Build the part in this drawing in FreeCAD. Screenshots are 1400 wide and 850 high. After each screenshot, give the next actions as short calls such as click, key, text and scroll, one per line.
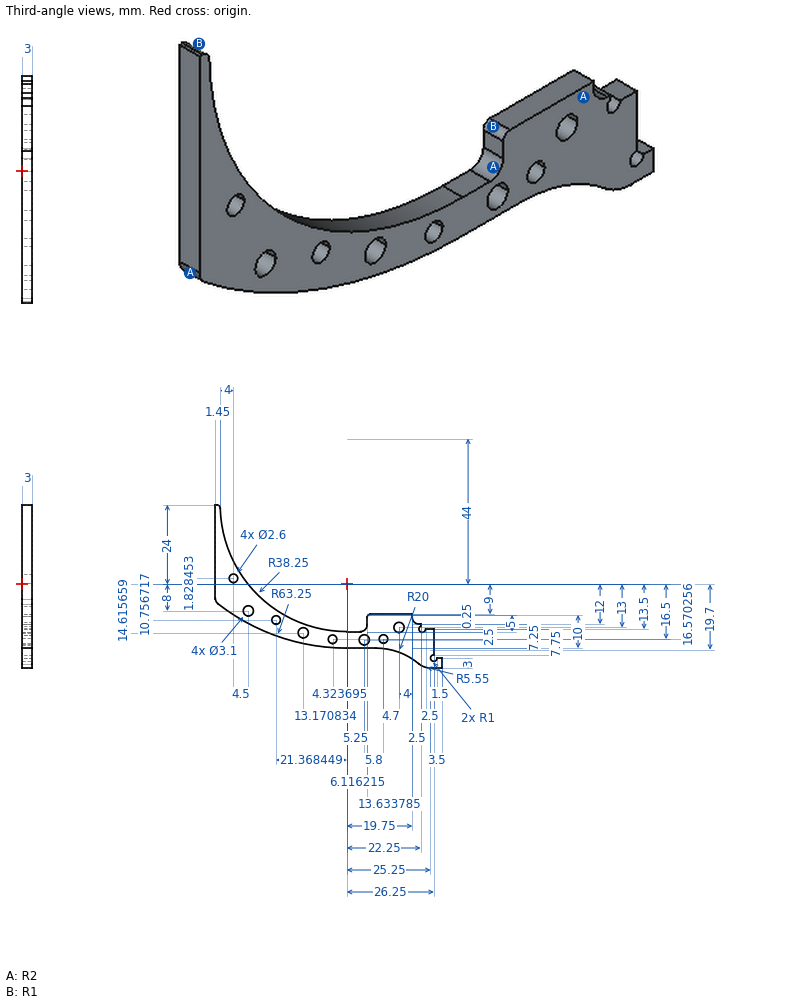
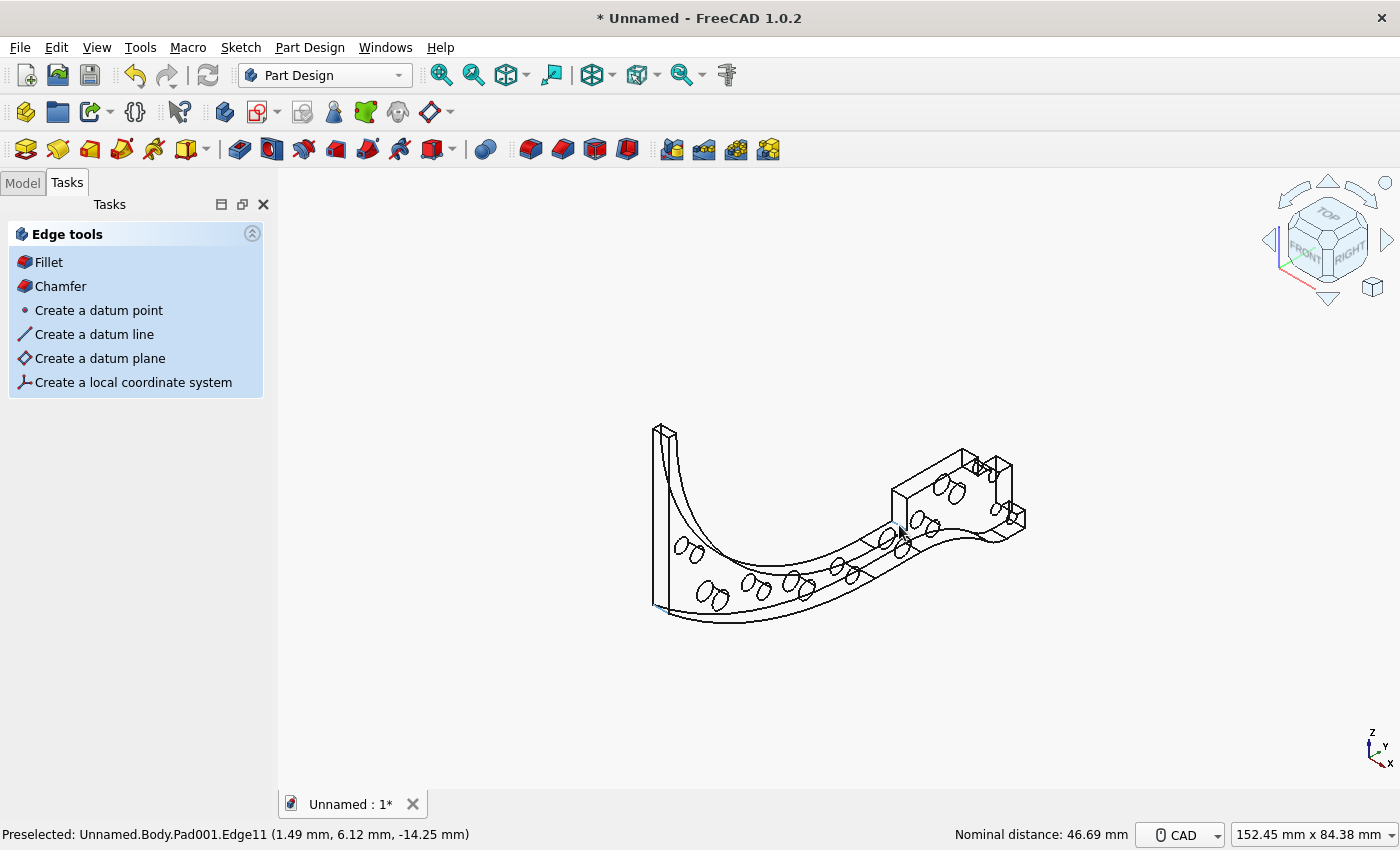
click(970, 470, ctrl)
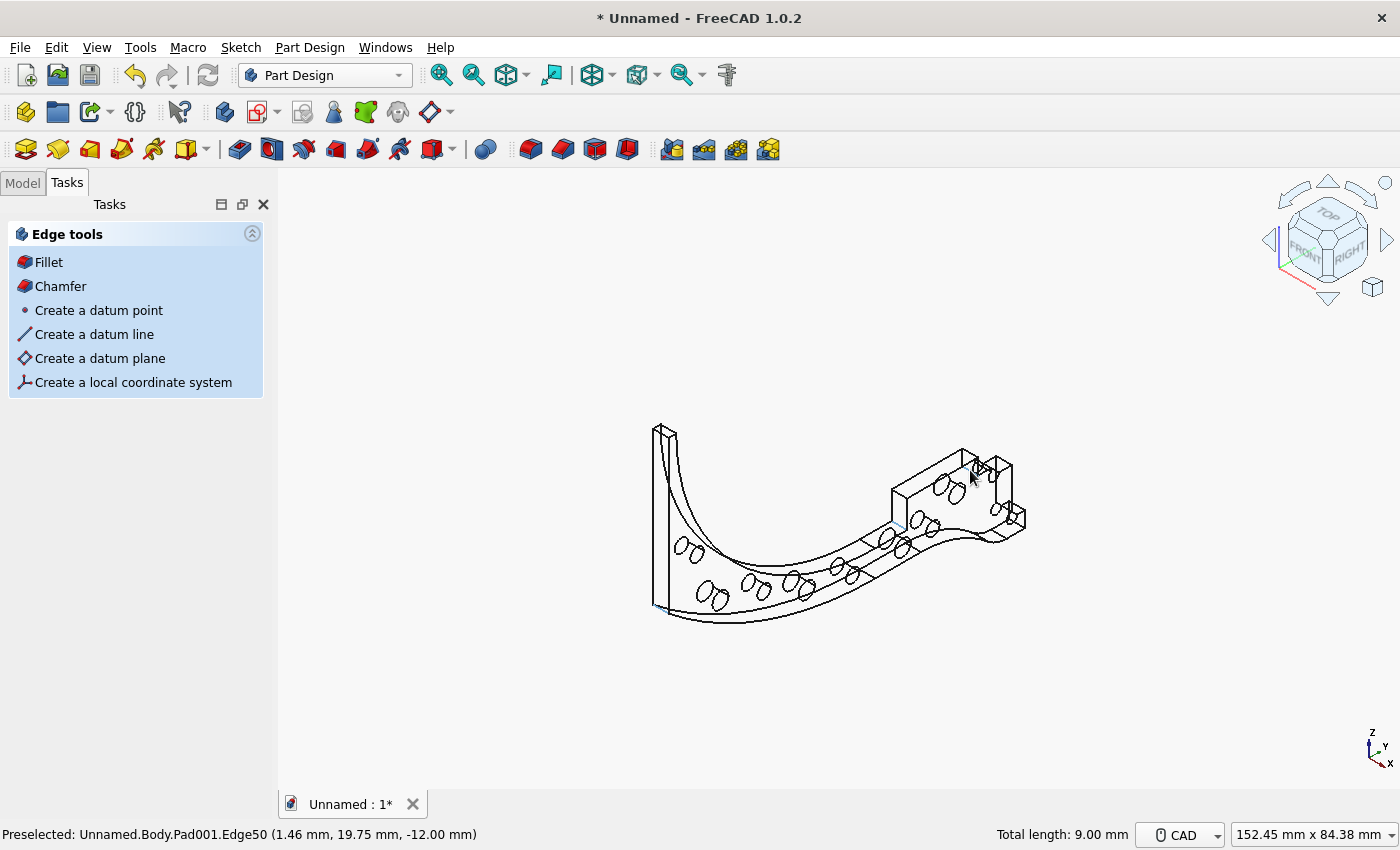
key(v)
key(1)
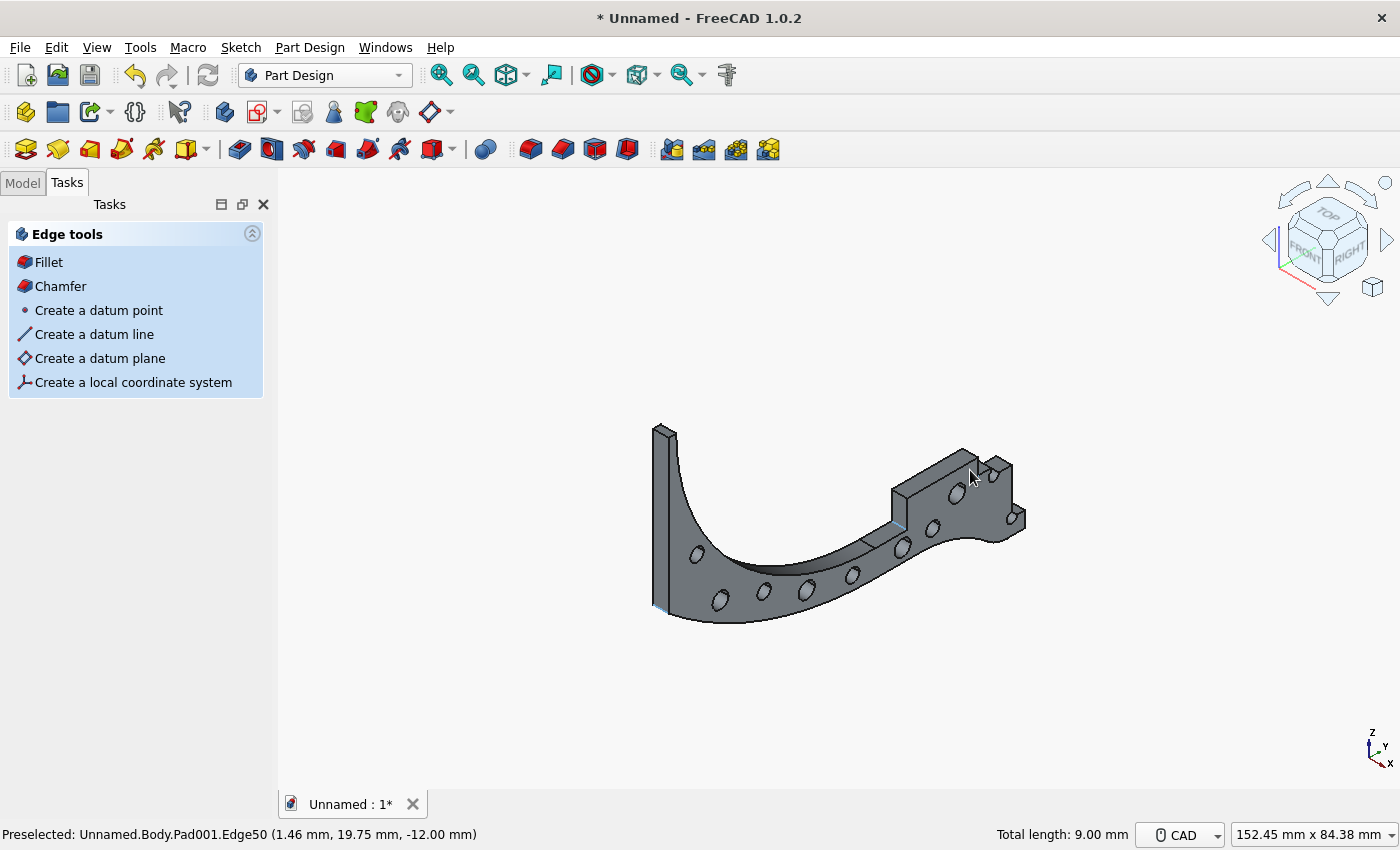
click(532, 150)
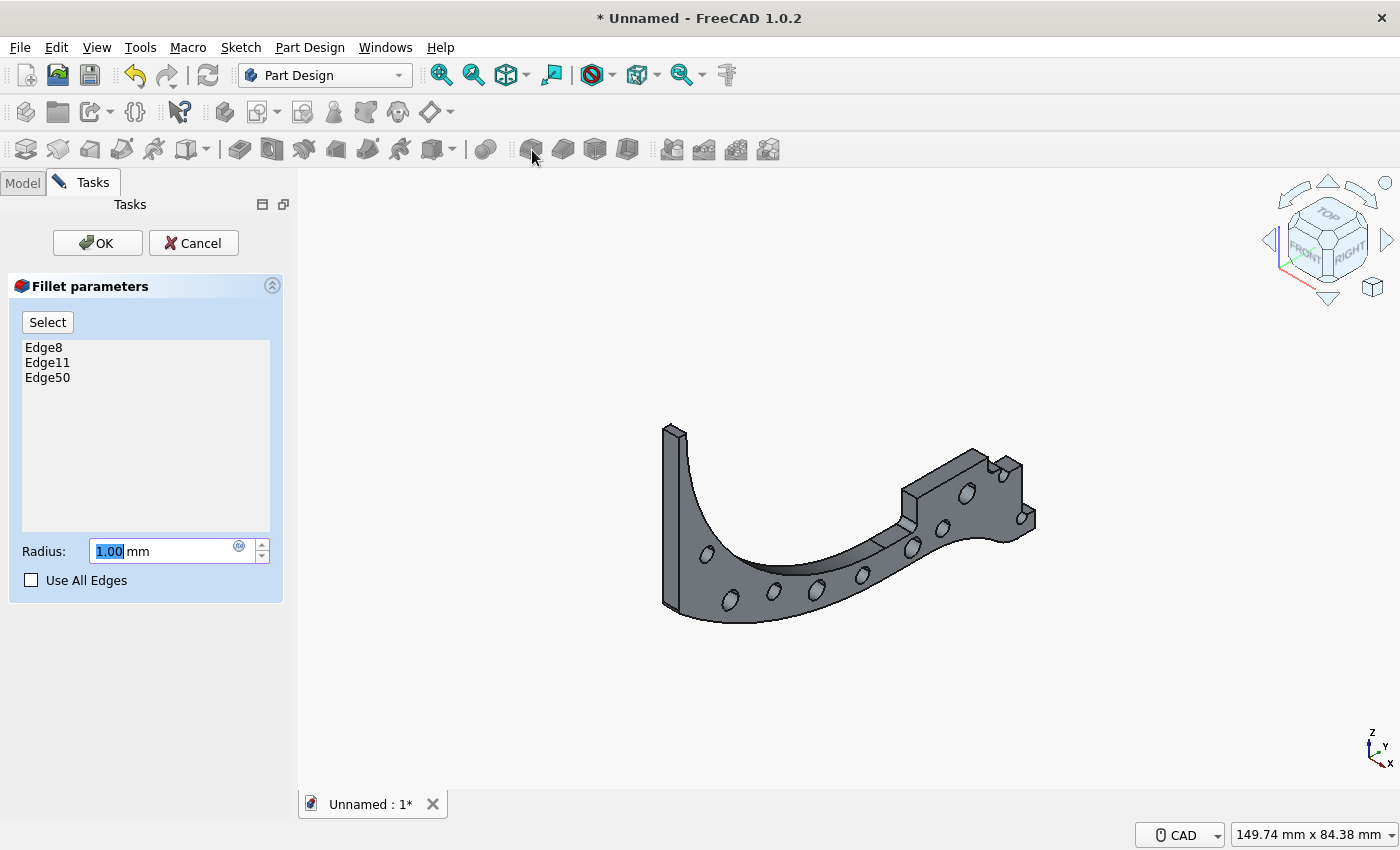
text(2)
key(Tab)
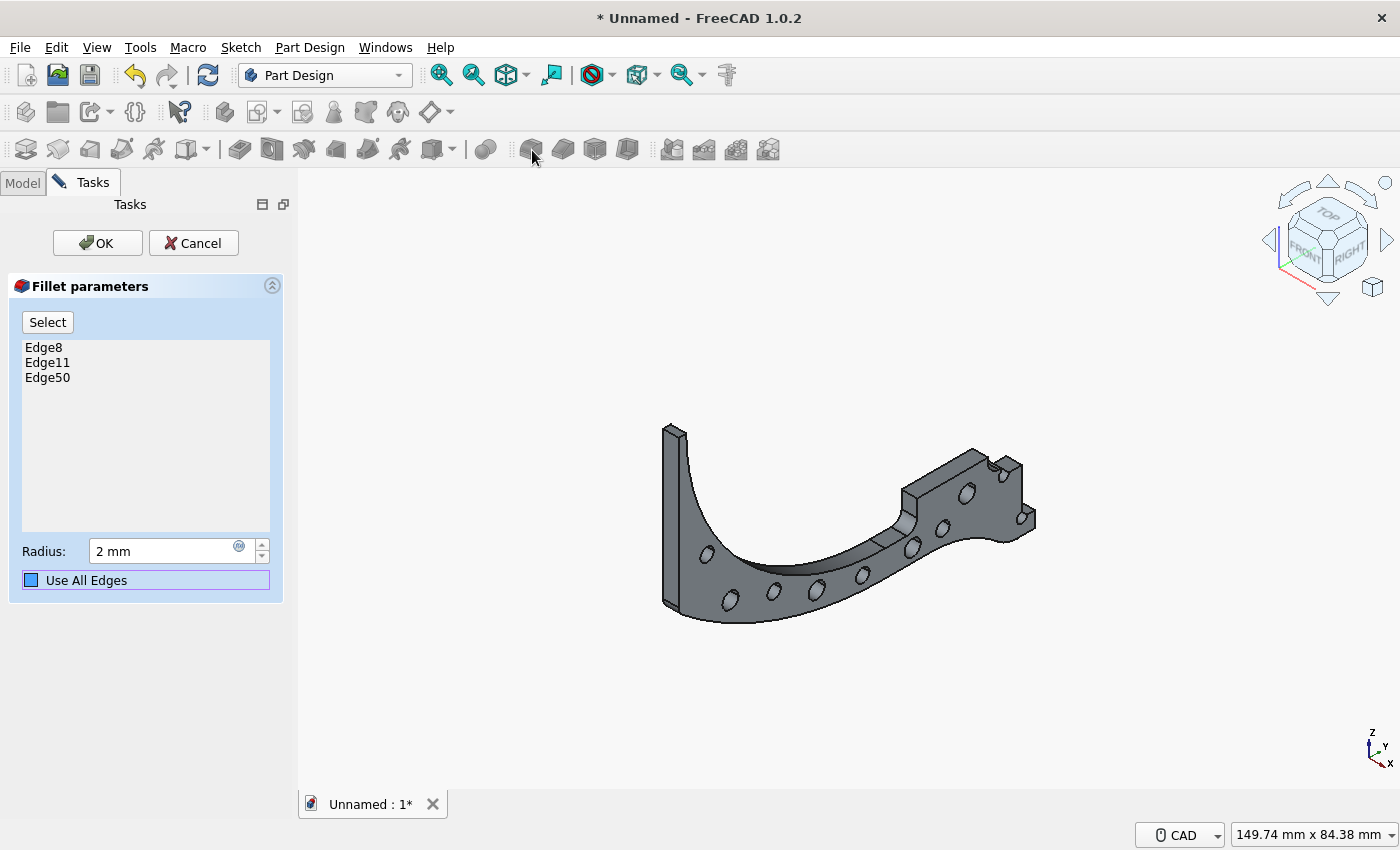
click(98, 243)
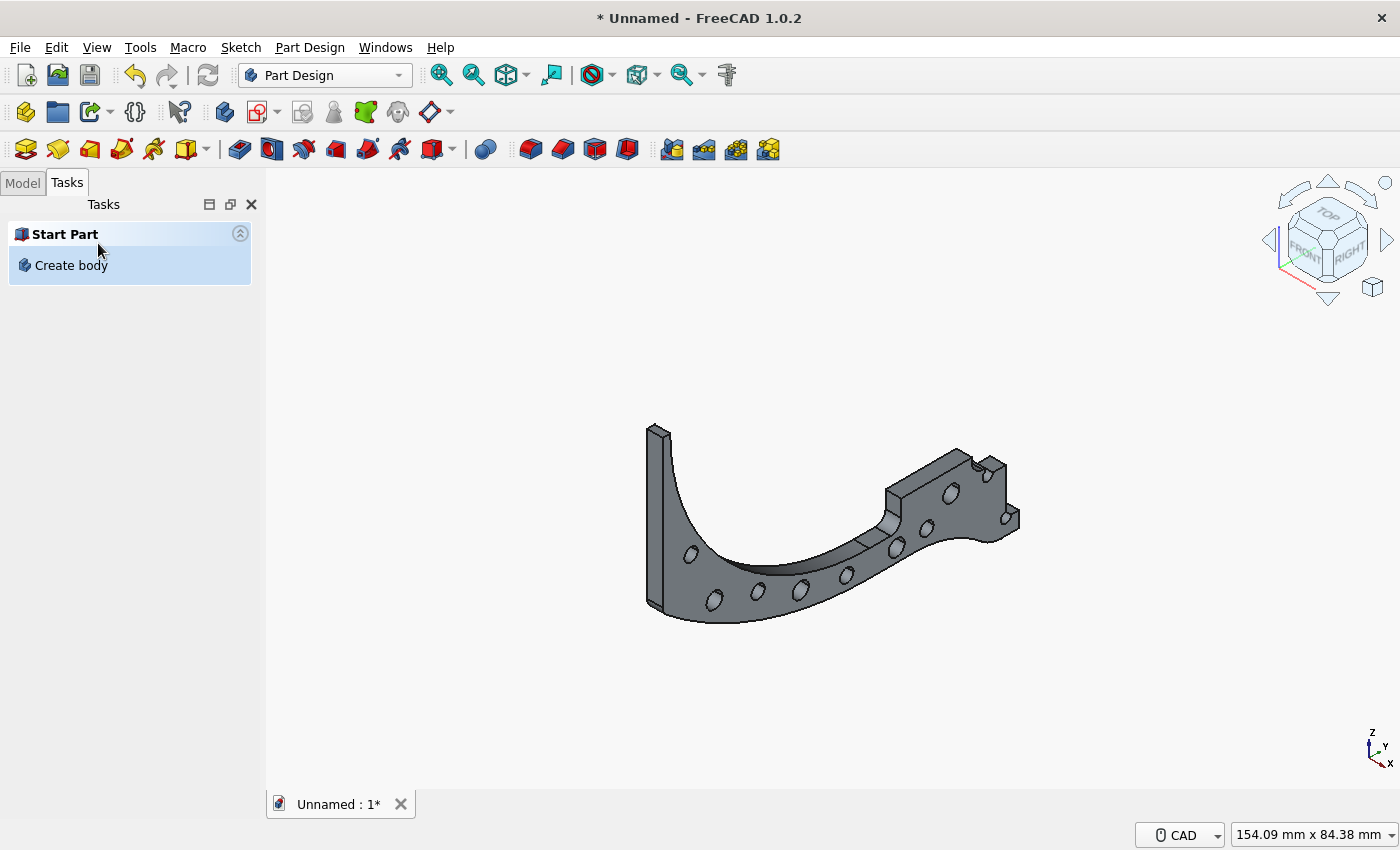
click(893, 493)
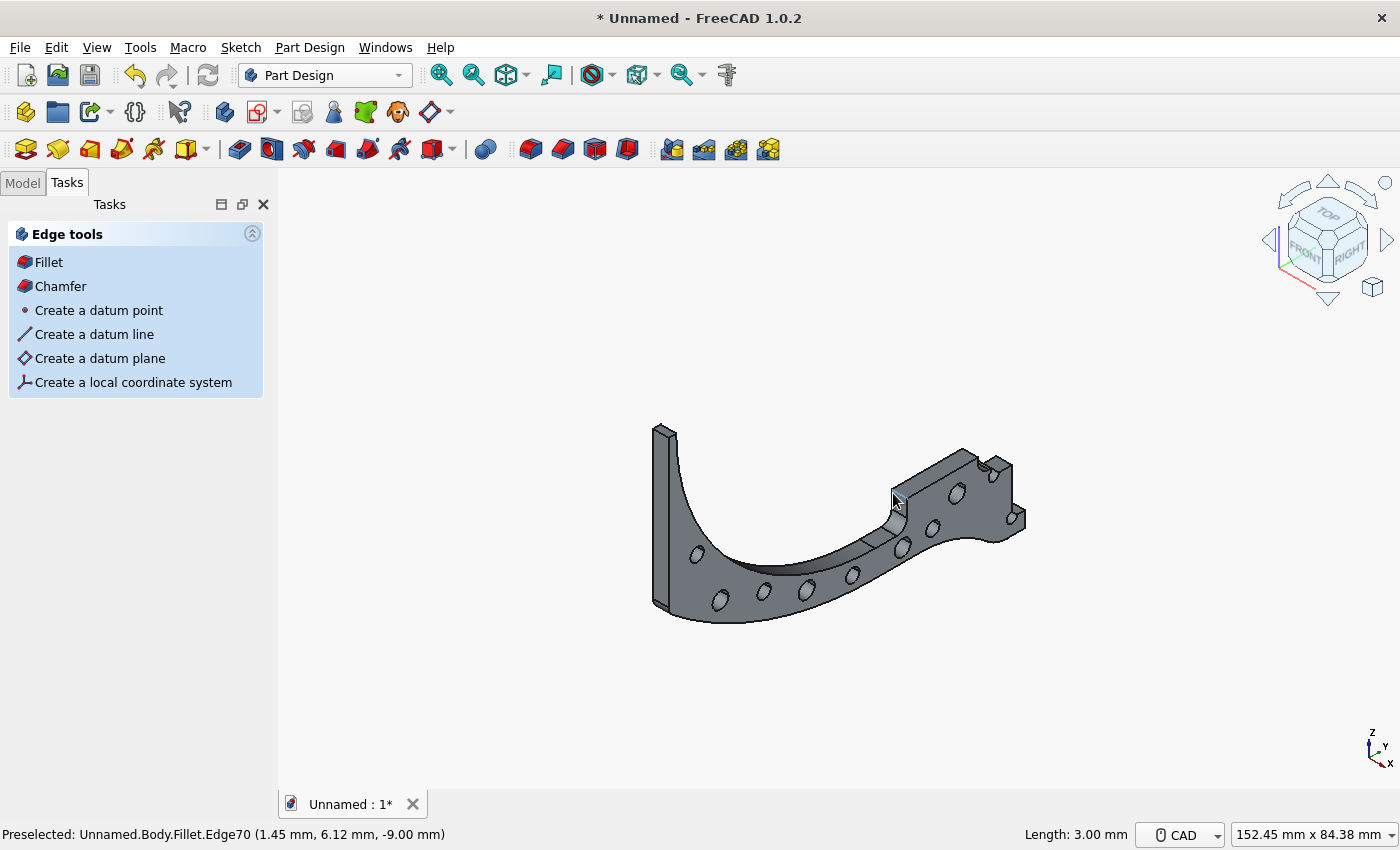
key(2)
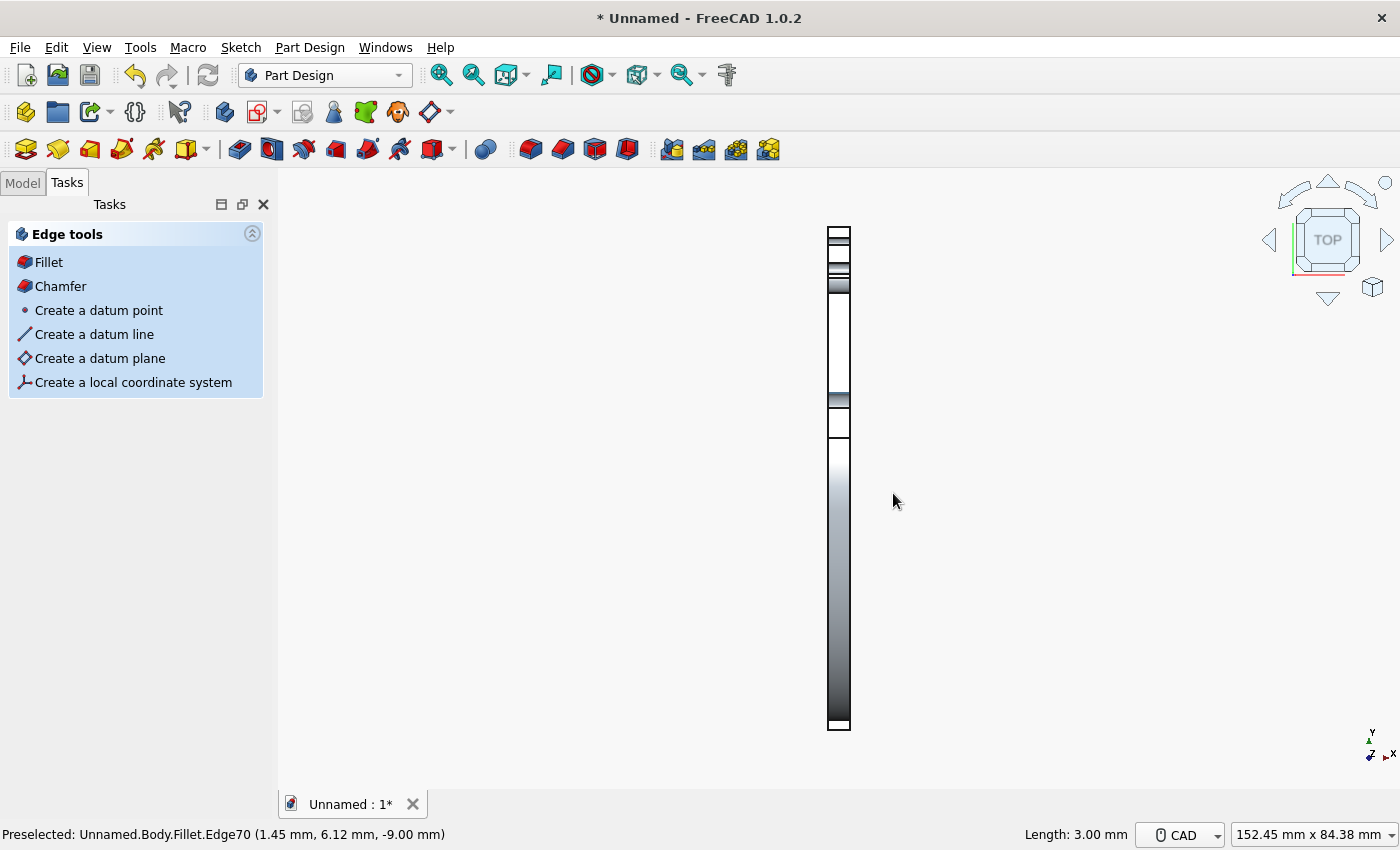
click(839, 719, ctrl)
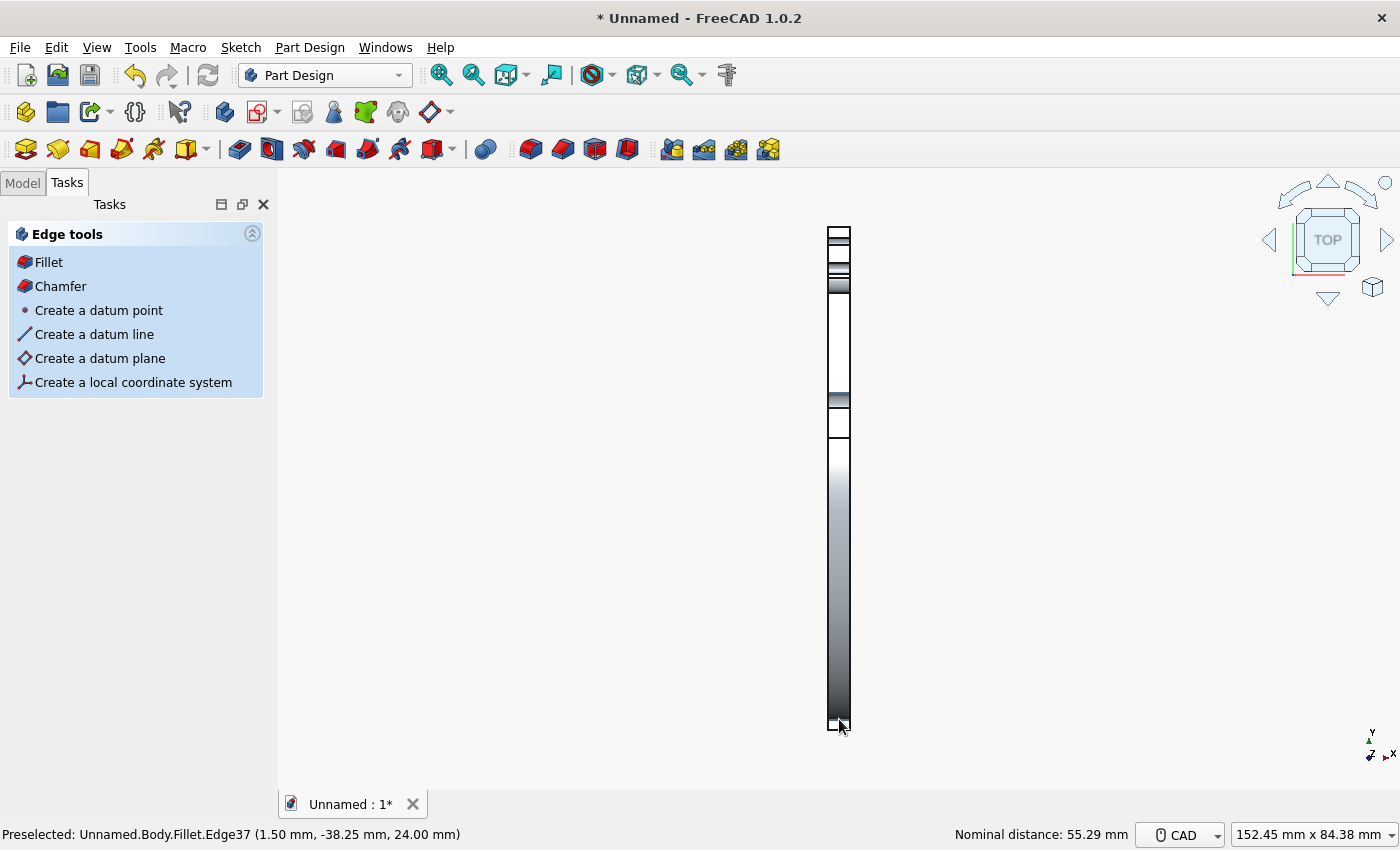
click(532, 150)